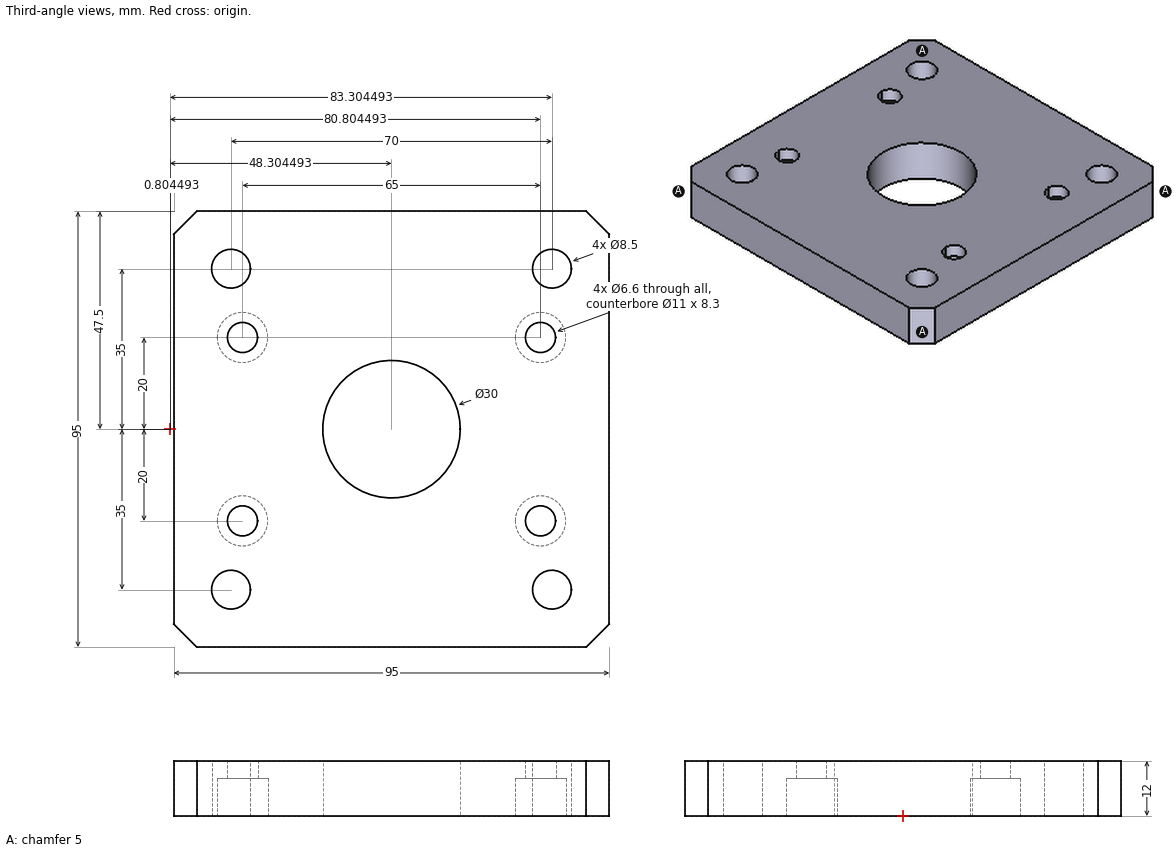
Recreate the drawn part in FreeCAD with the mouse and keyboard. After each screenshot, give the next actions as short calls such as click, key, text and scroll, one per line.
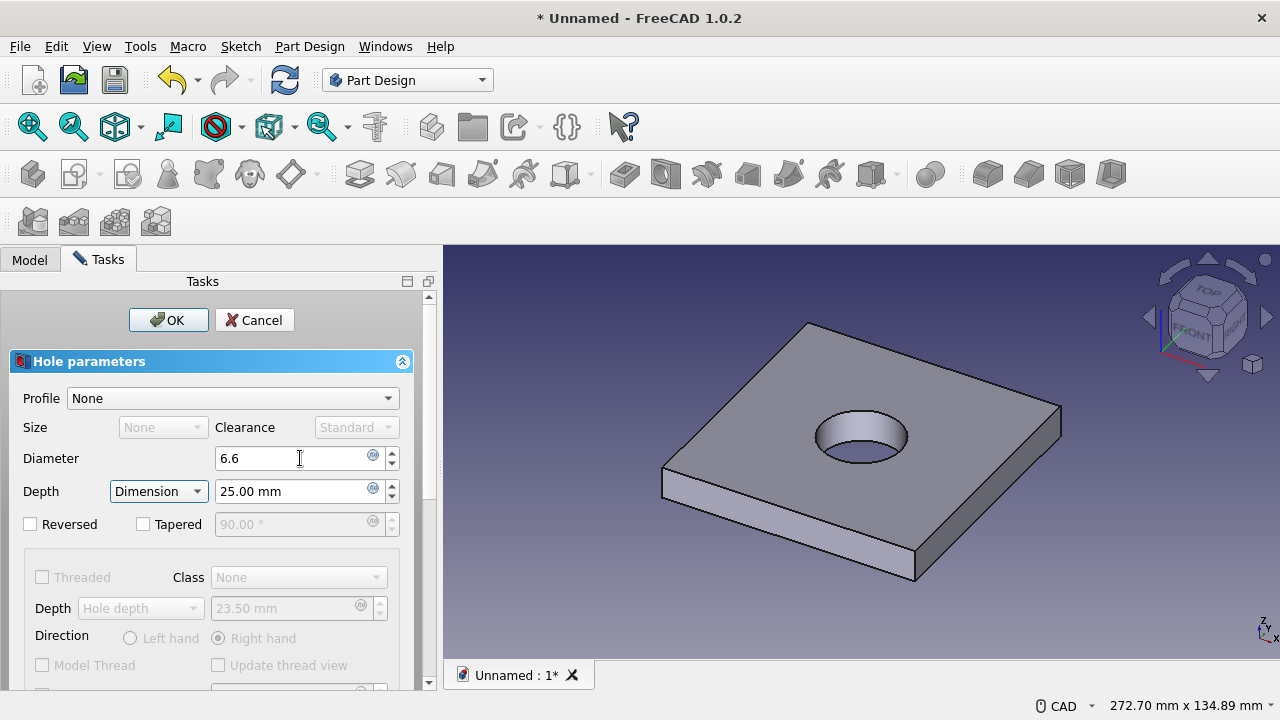
click(160, 492)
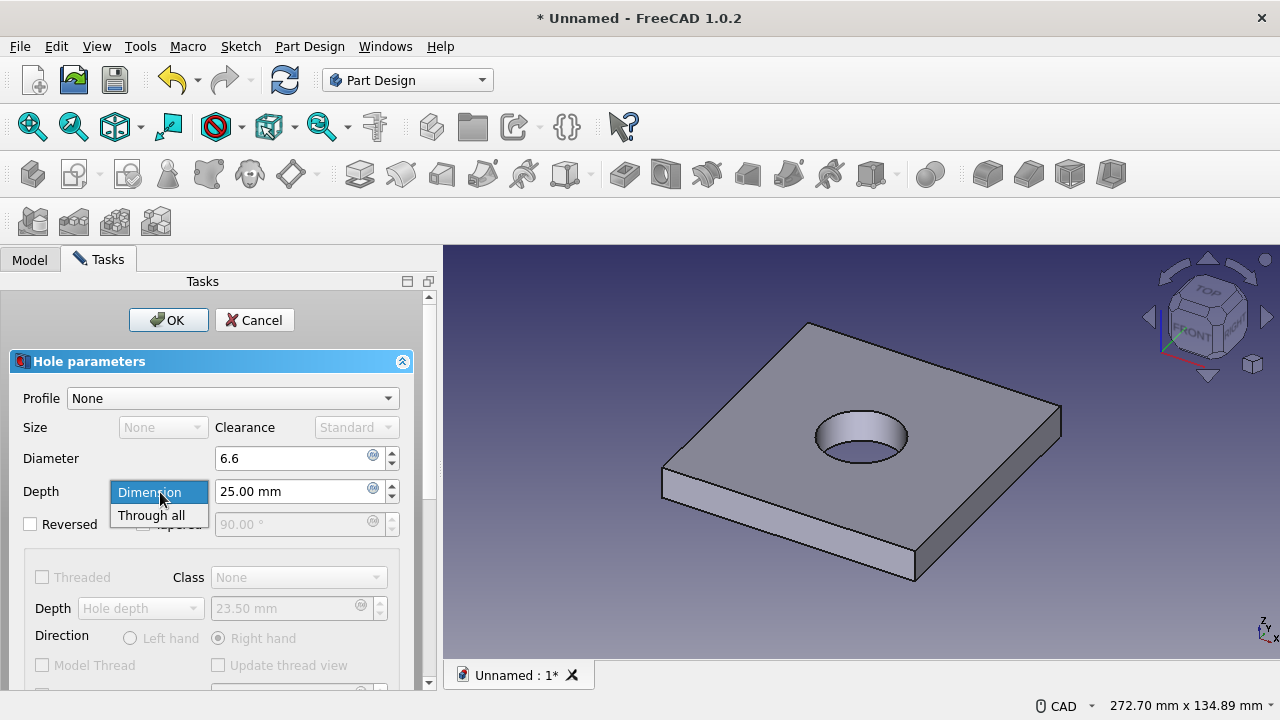
click(158, 516)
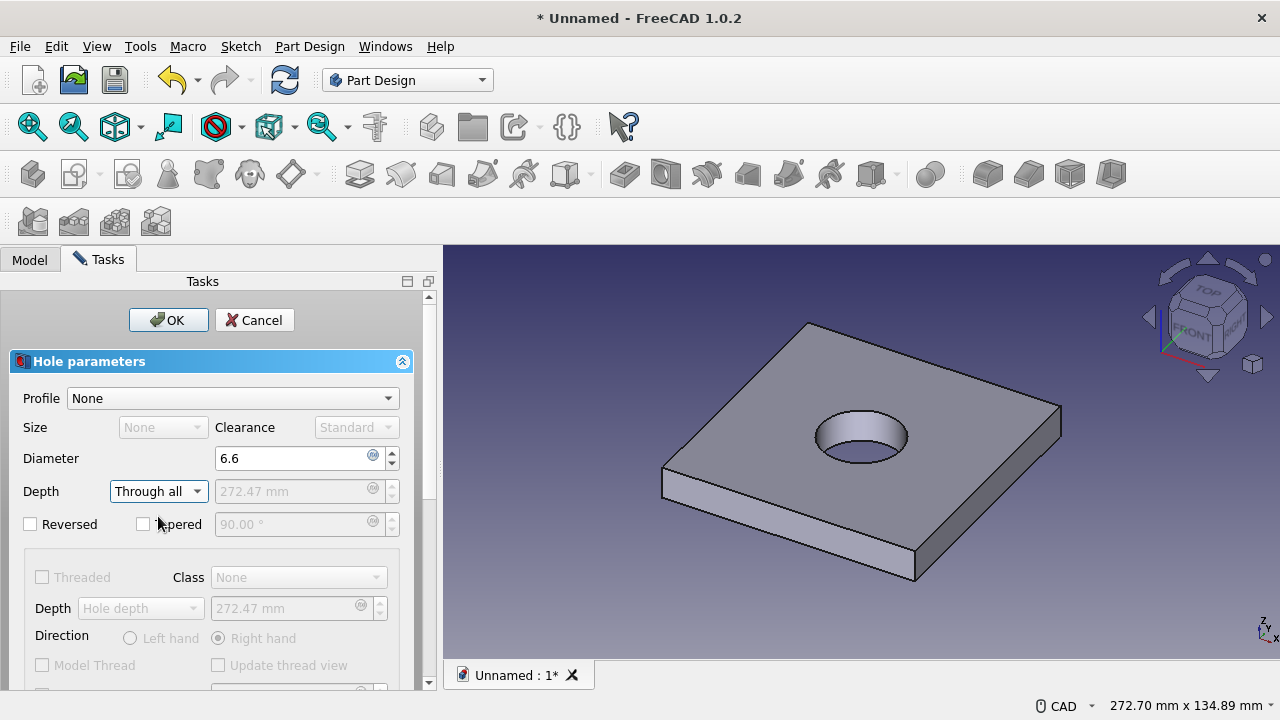
click(31, 524)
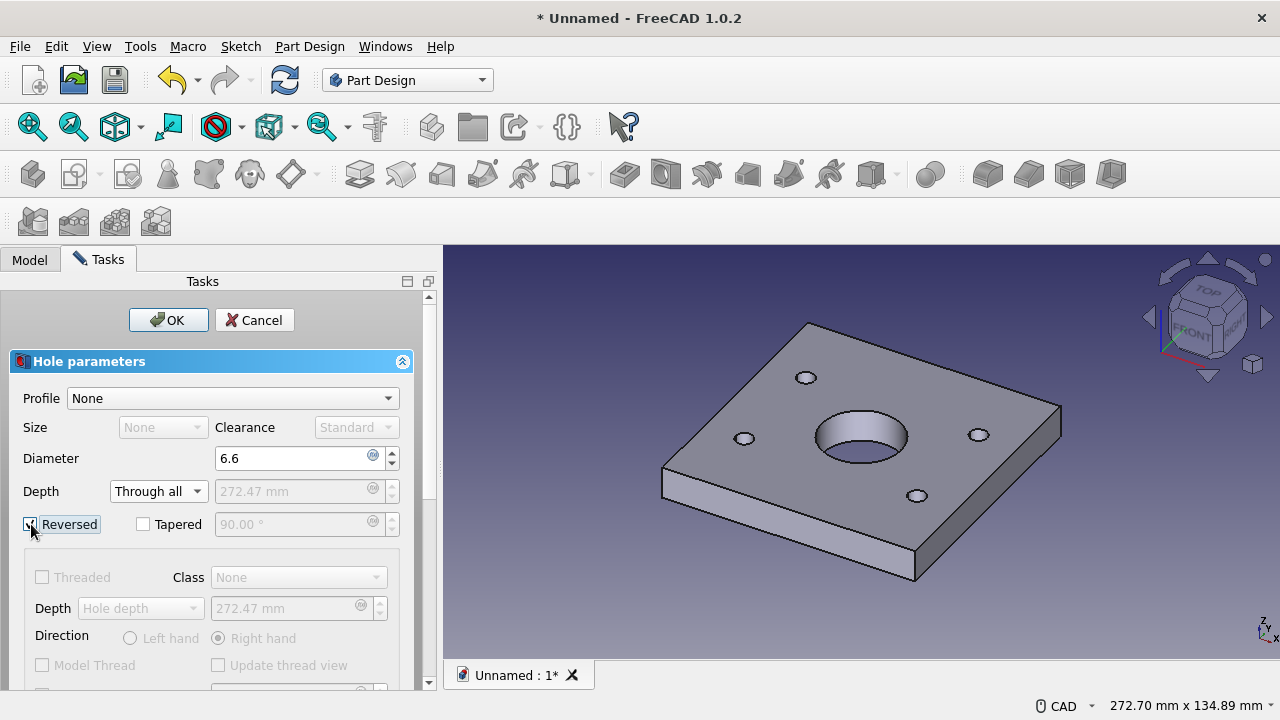
scroll(429, 490, down, 3)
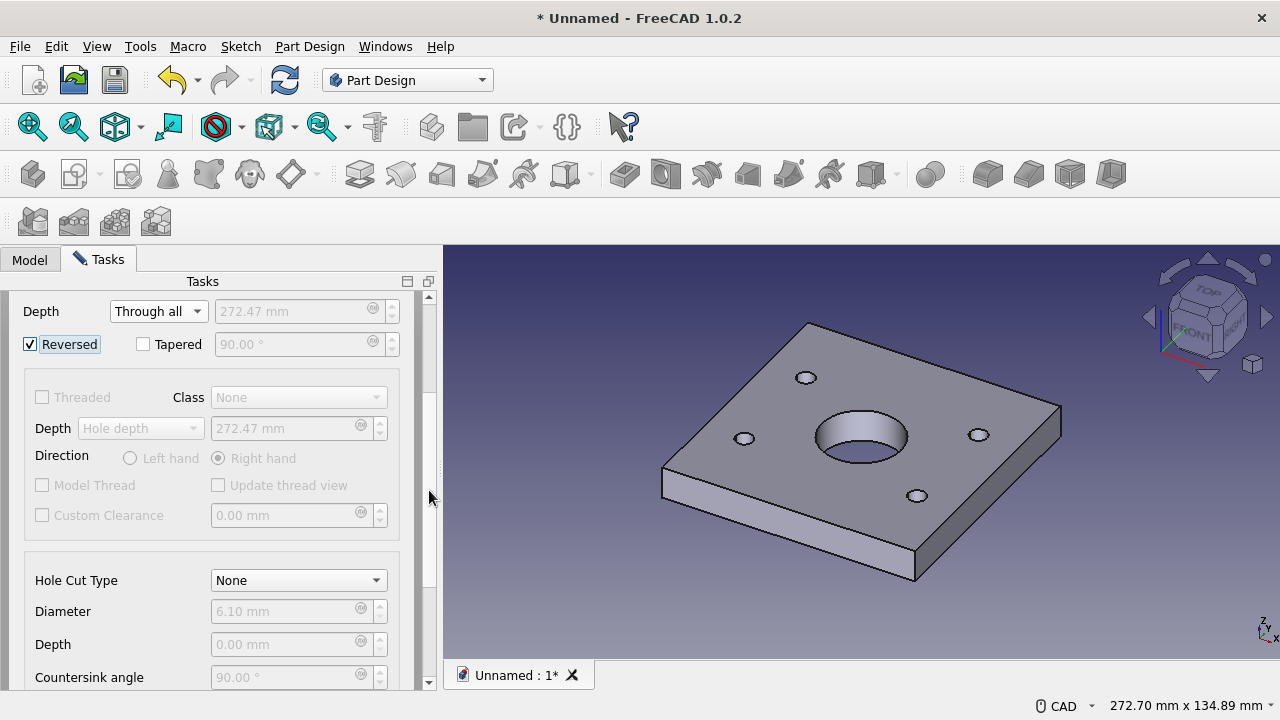
click(300, 580)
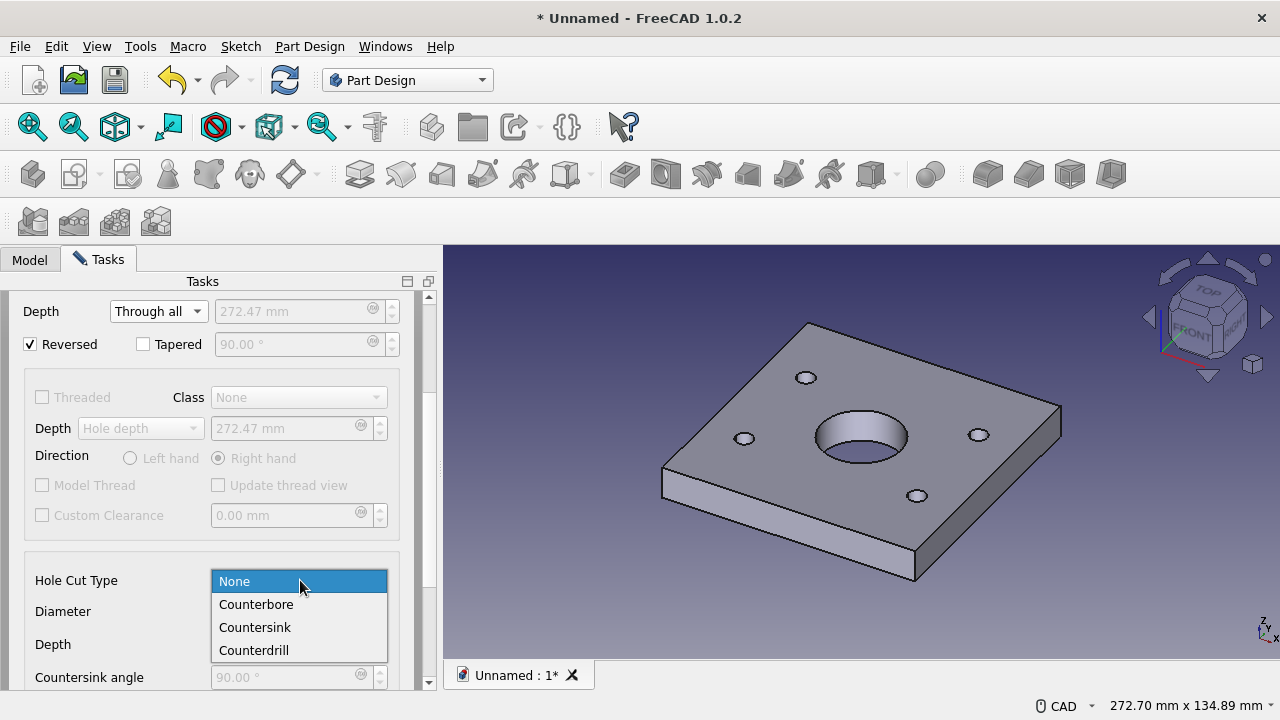
click(298, 604)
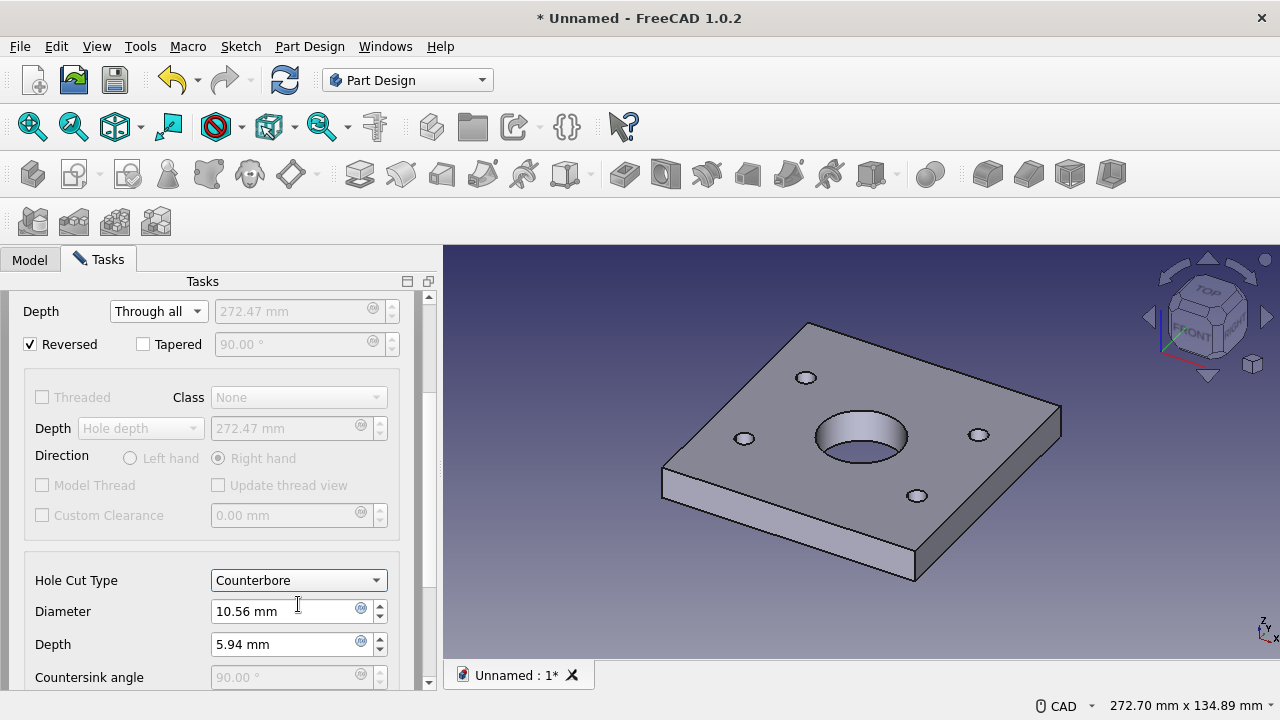
triple_click(292, 612)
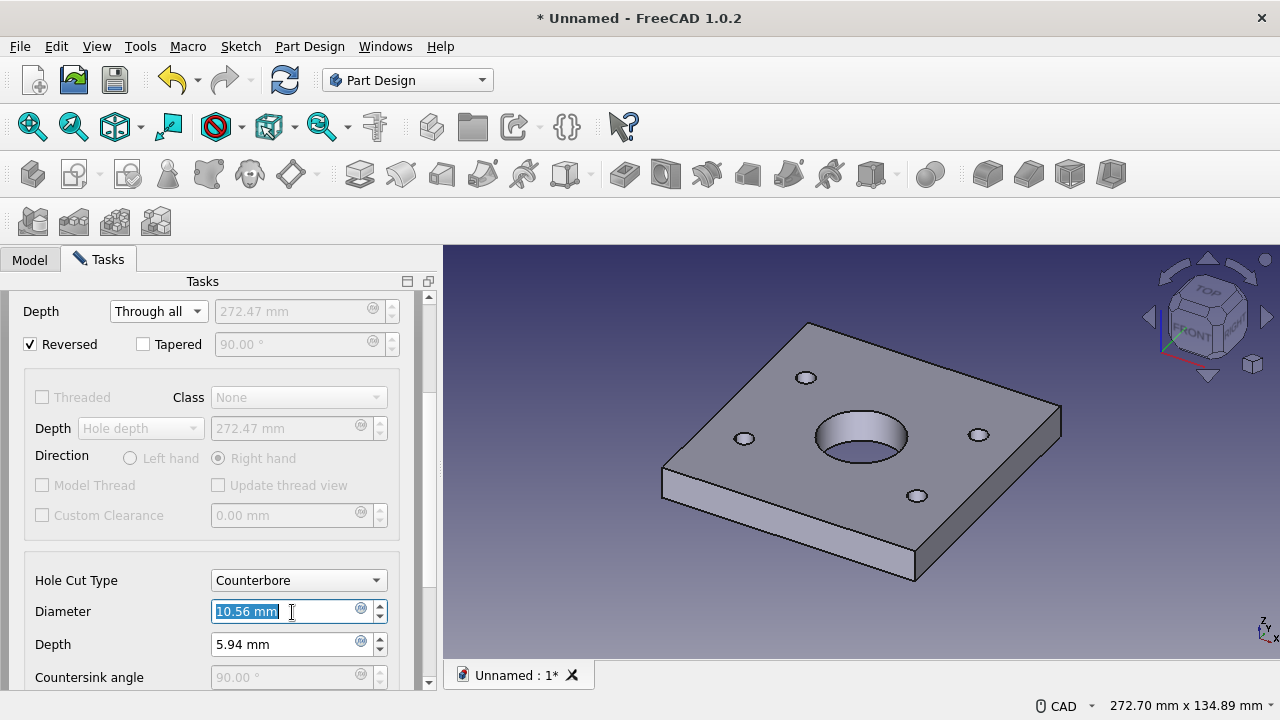
text(11)
key(Tab)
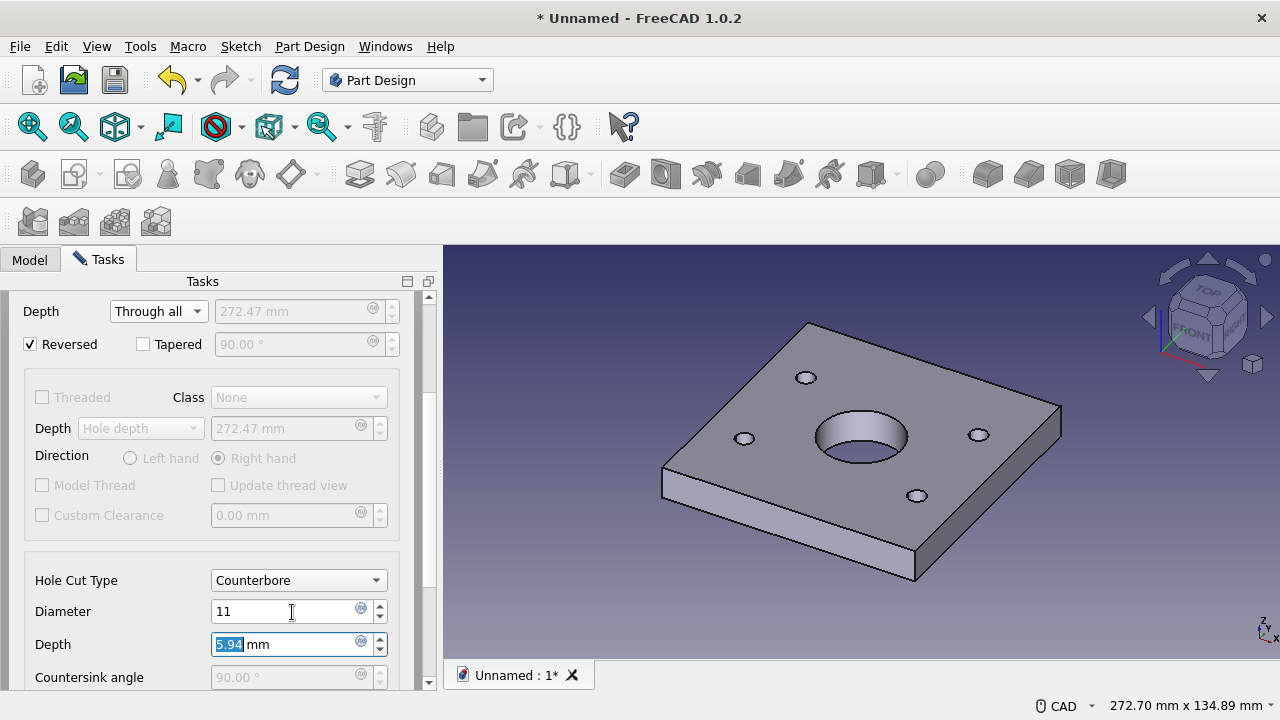
text(8.3)
key(Tab)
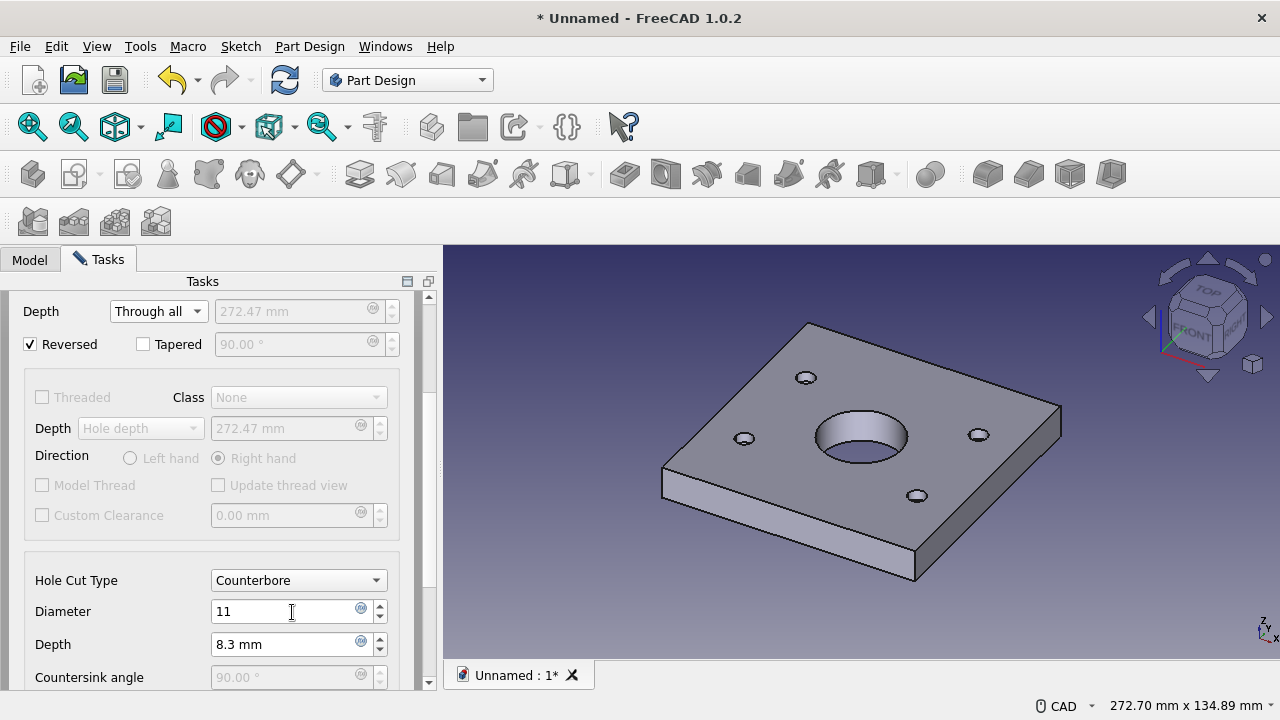
scroll(429, 490, up, 4)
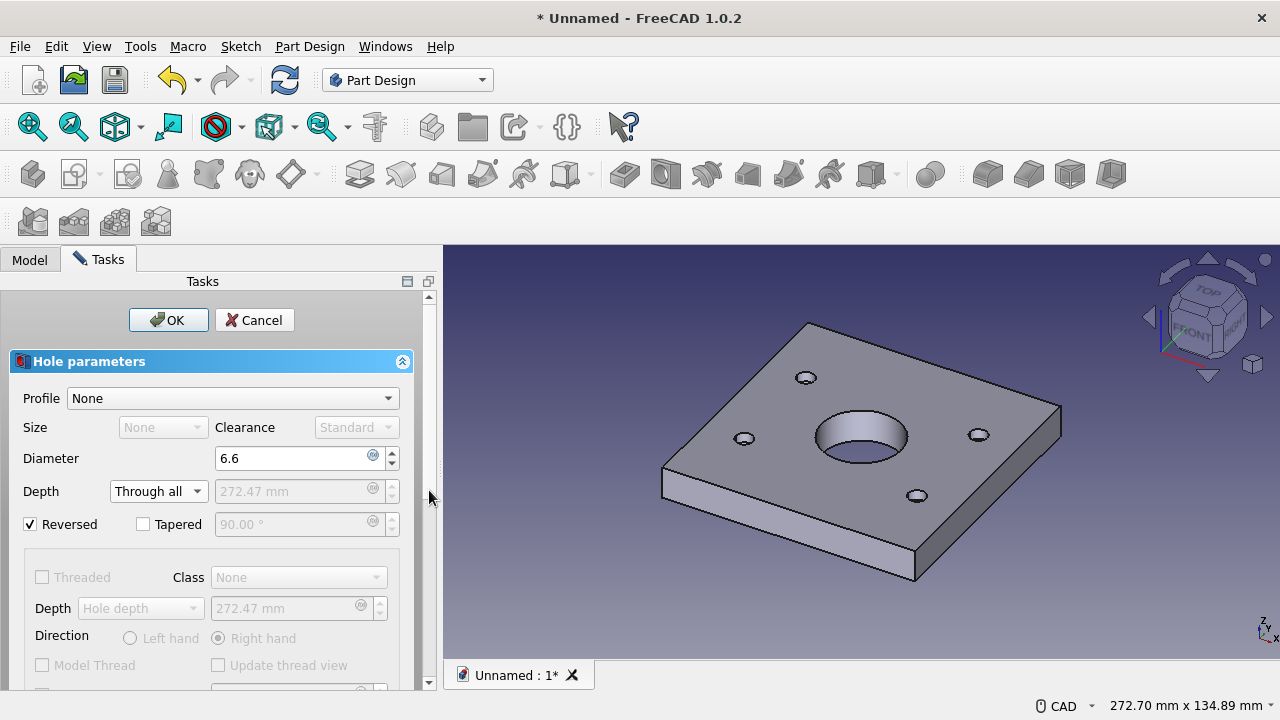
click(169, 320)